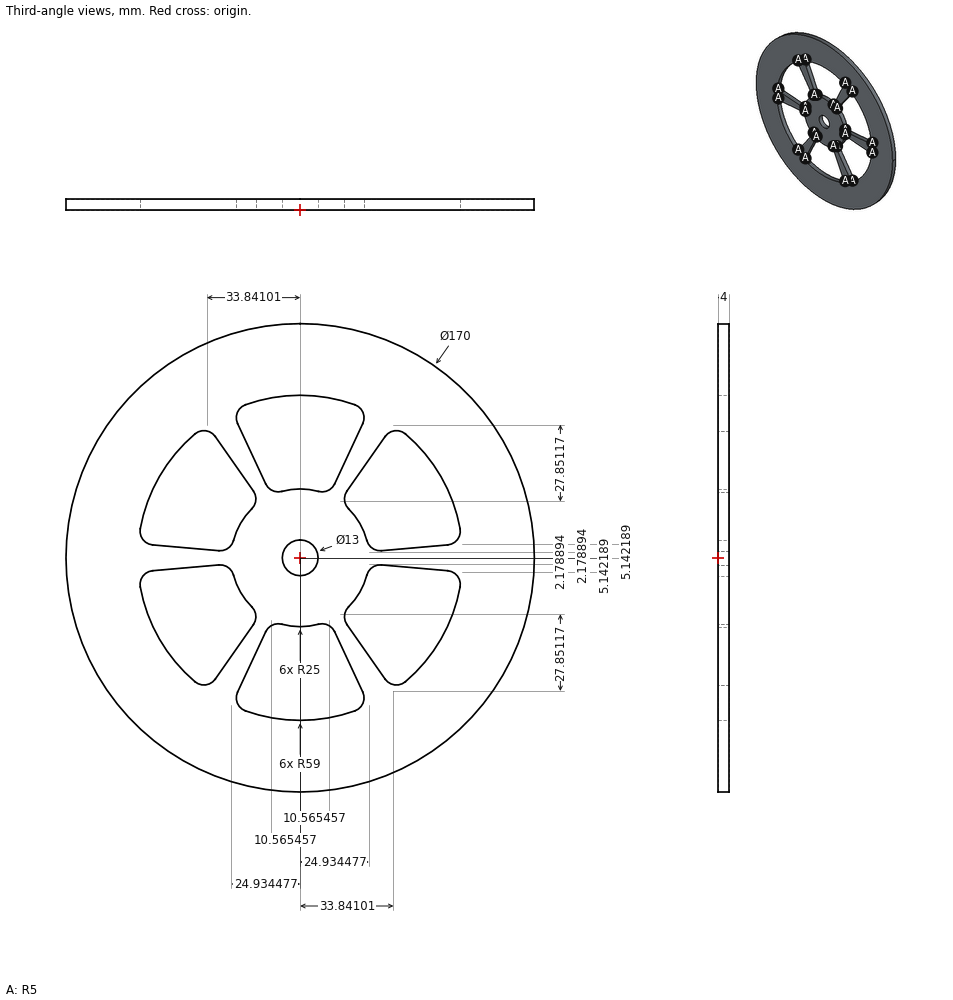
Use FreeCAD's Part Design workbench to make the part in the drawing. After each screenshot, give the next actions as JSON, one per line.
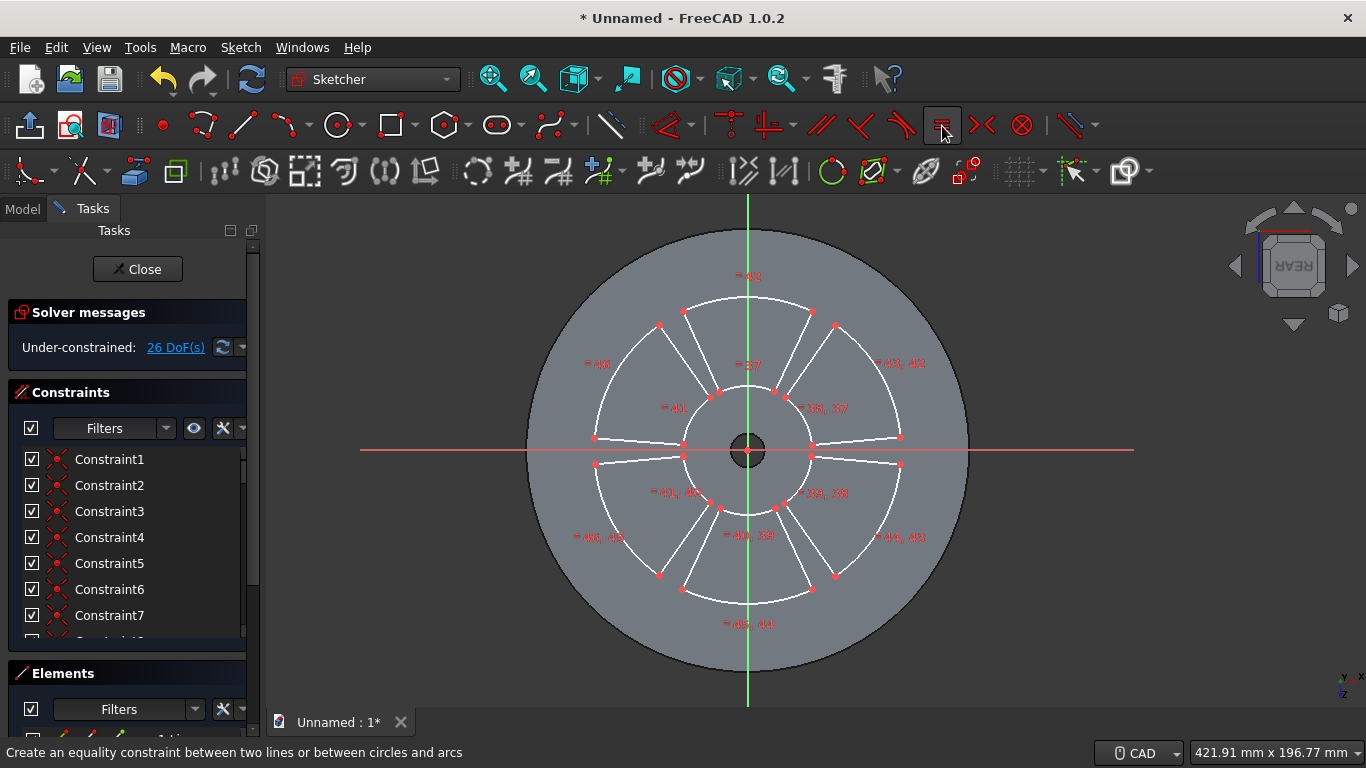
{"action": "left_click", "coordinate": [666, 126]}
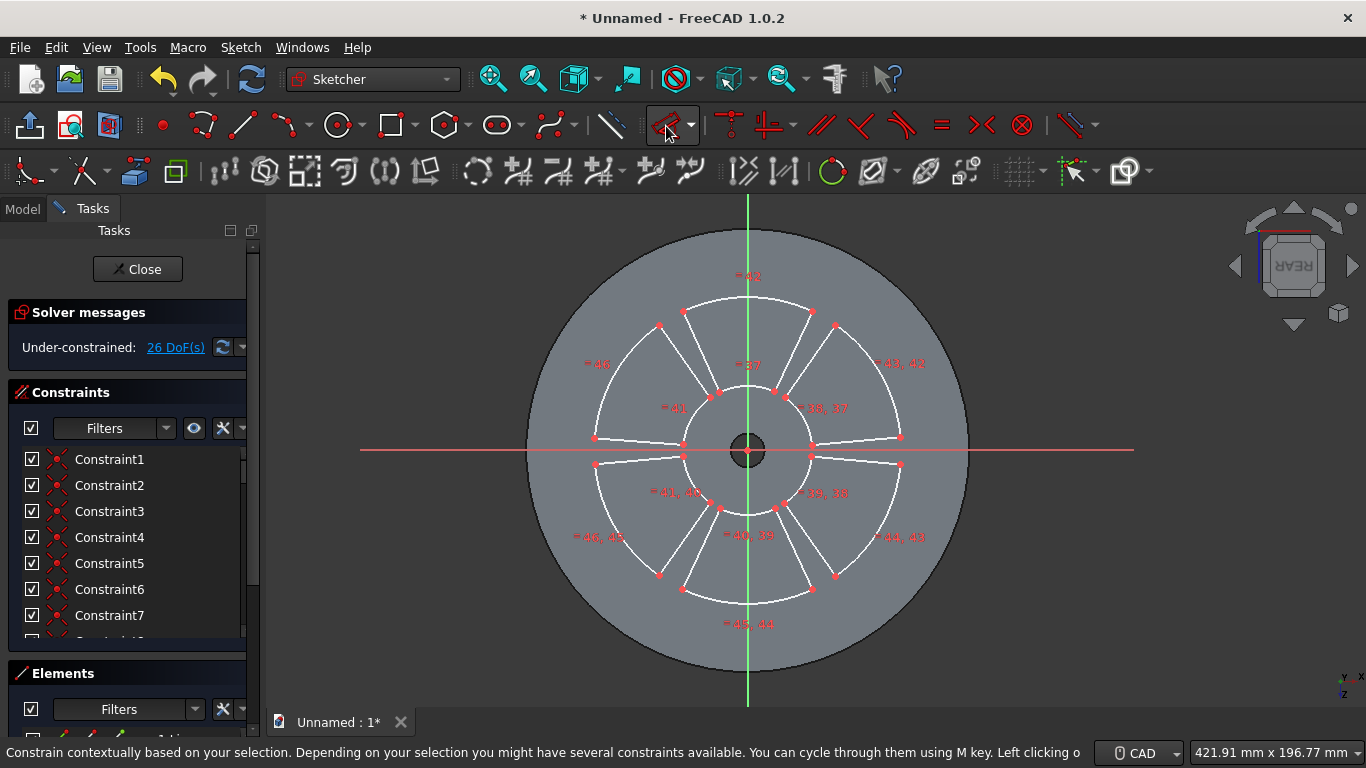
{"action": "left_click", "coordinate": [775, 300]}
{"action": "left_click", "coordinate": [781, 269]}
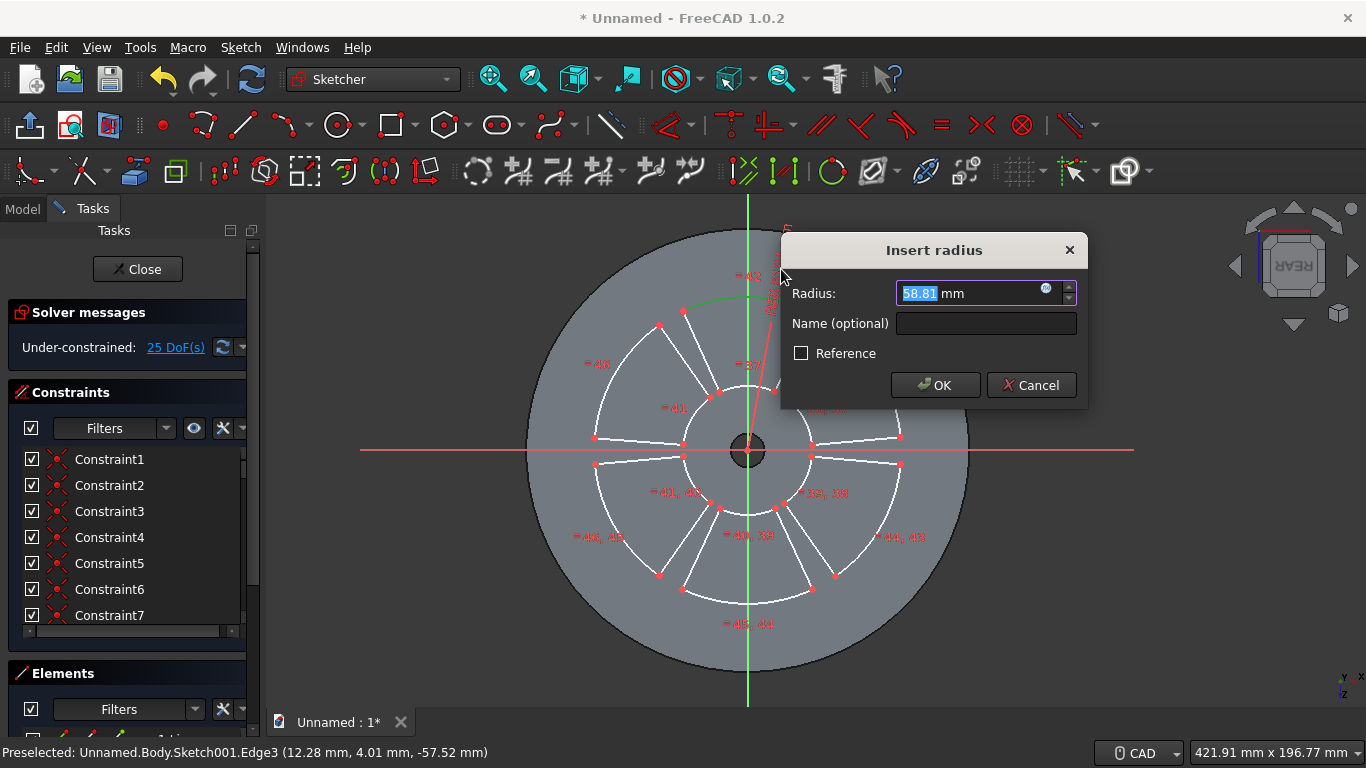
{"action": "type", "text": "59"}
{"action": "key", "text": "Return"}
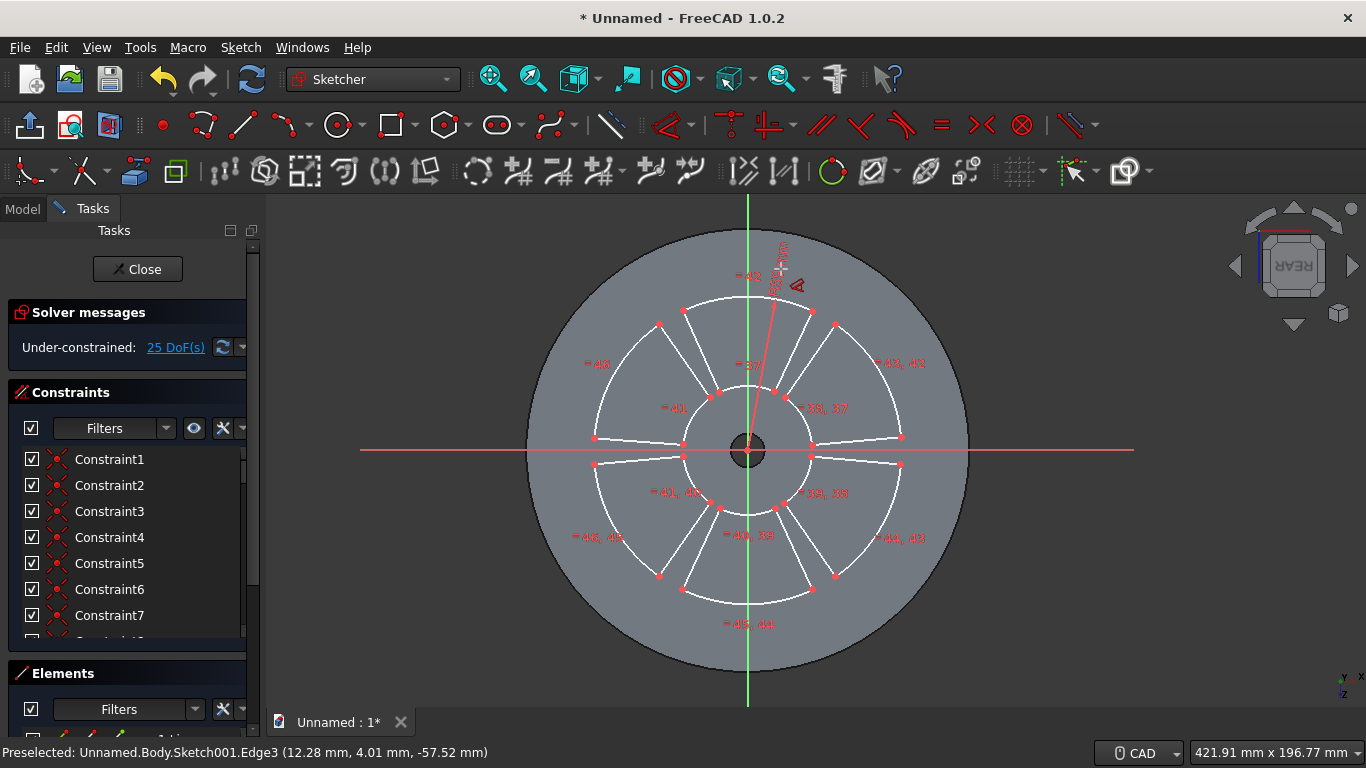
{"action": "scroll", "coordinate": [759, 387], "scroll_direction": "up", "scroll_amount": 2}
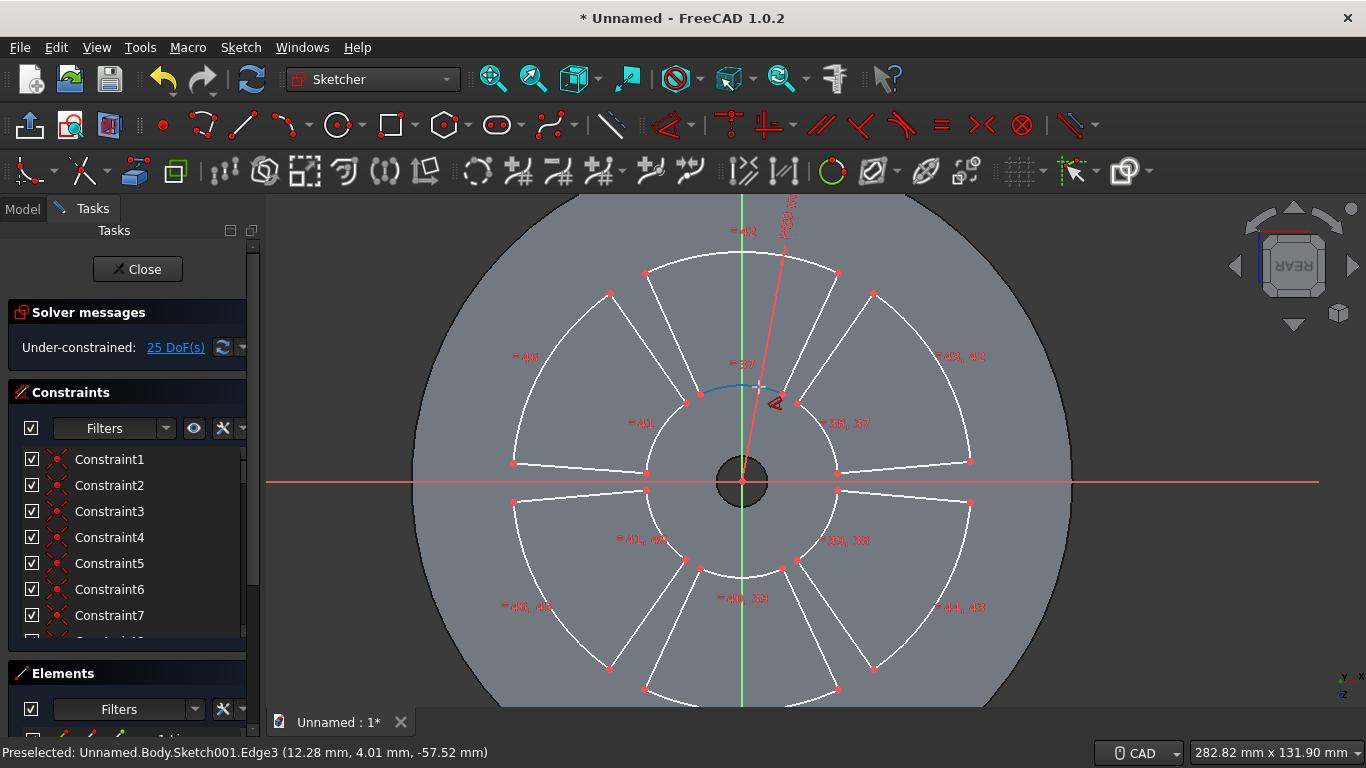
{"action": "left_click", "coordinate": [758, 387]}
{"action": "left_click", "coordinate": [763, 355]}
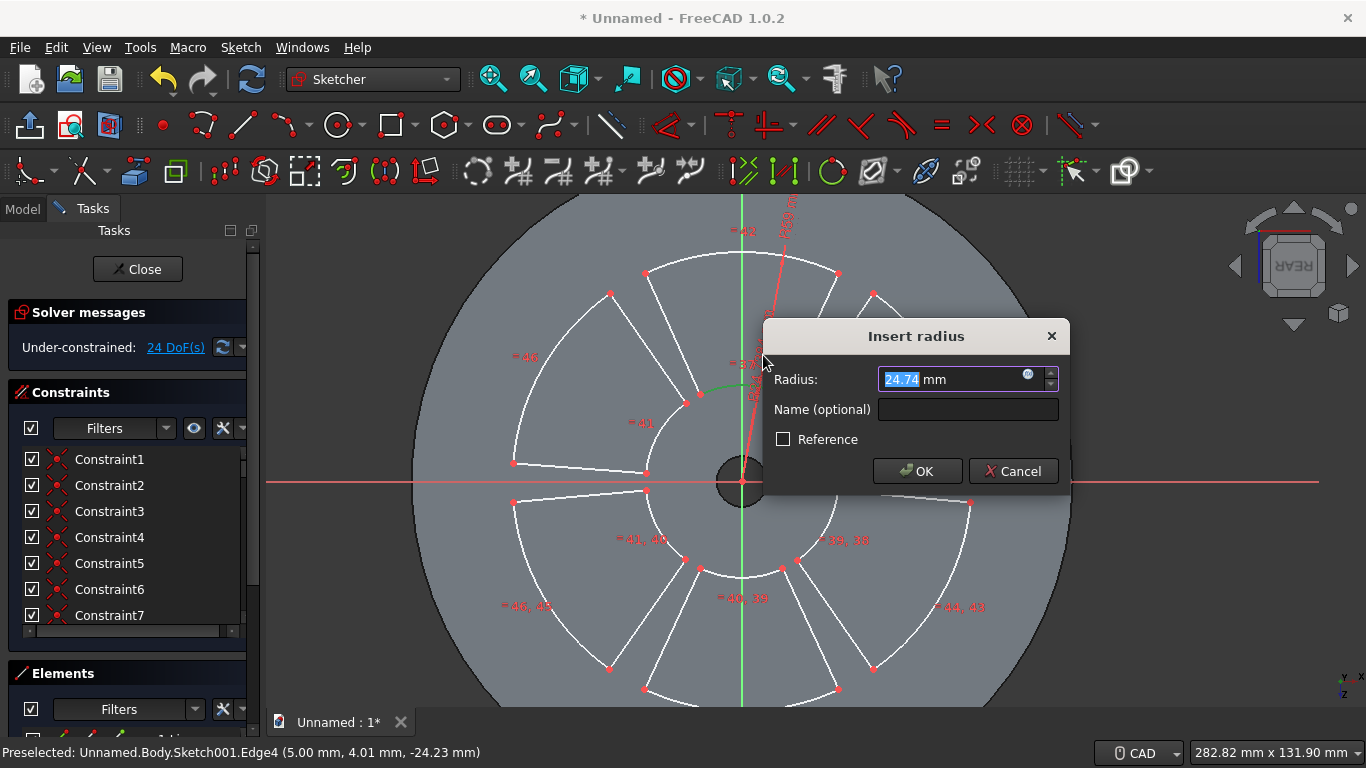
{"action": "type", "text": "25"}
{"action": "key", "text": "Return"}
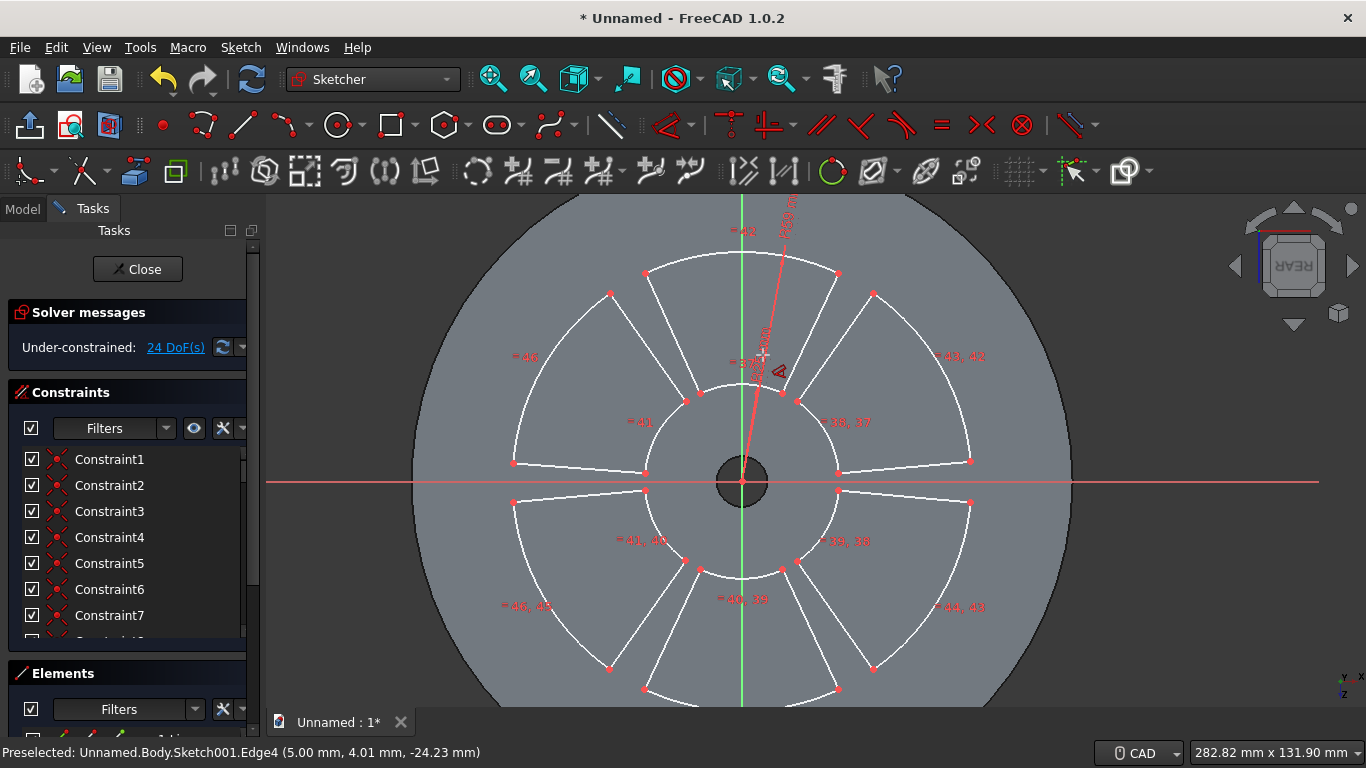
{"action": "left_click", "coordinate": [874, 294]}
{"action": "left_click", "coordinate": [854, 260]}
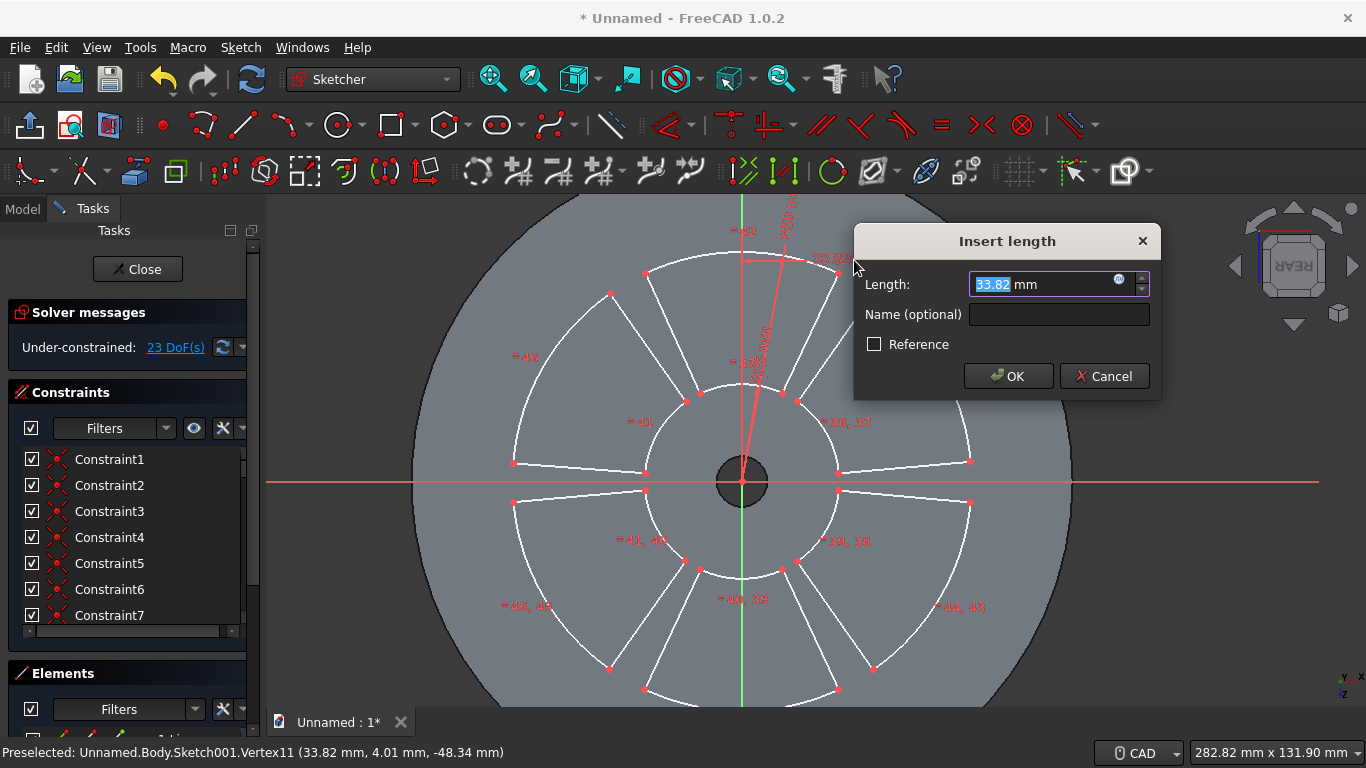
{"action": "type", "text": "33.84101"}
{"action": "key", "text": "Return"}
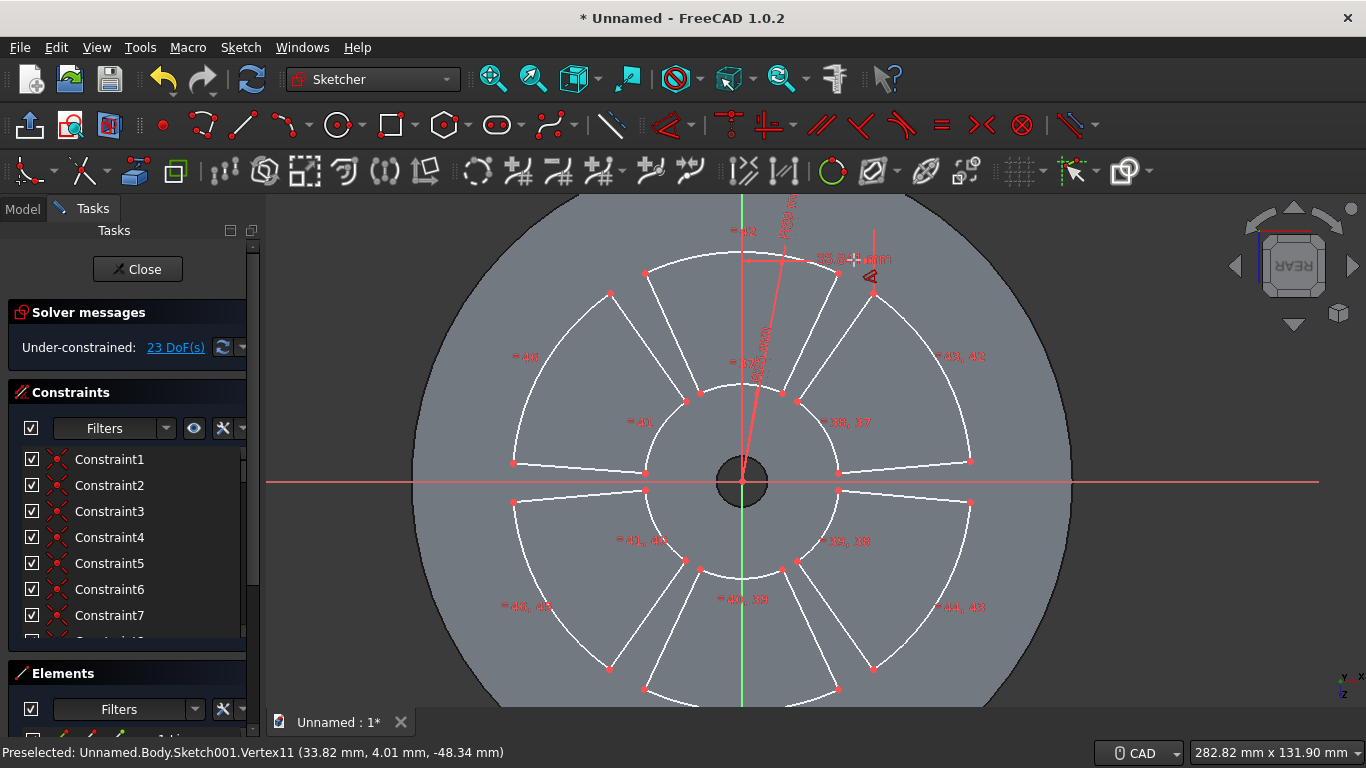
{"action": "scroll", "coordinate": [839, 473], "scroll_direction": "up", "scroll_amount": 8}